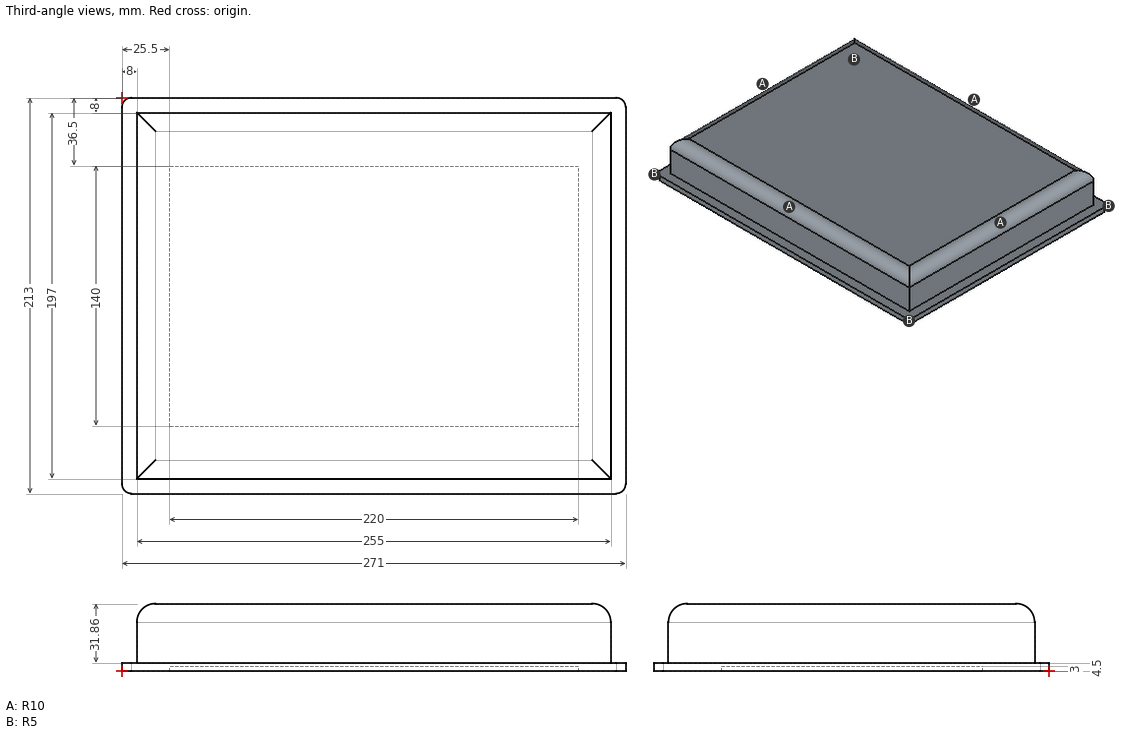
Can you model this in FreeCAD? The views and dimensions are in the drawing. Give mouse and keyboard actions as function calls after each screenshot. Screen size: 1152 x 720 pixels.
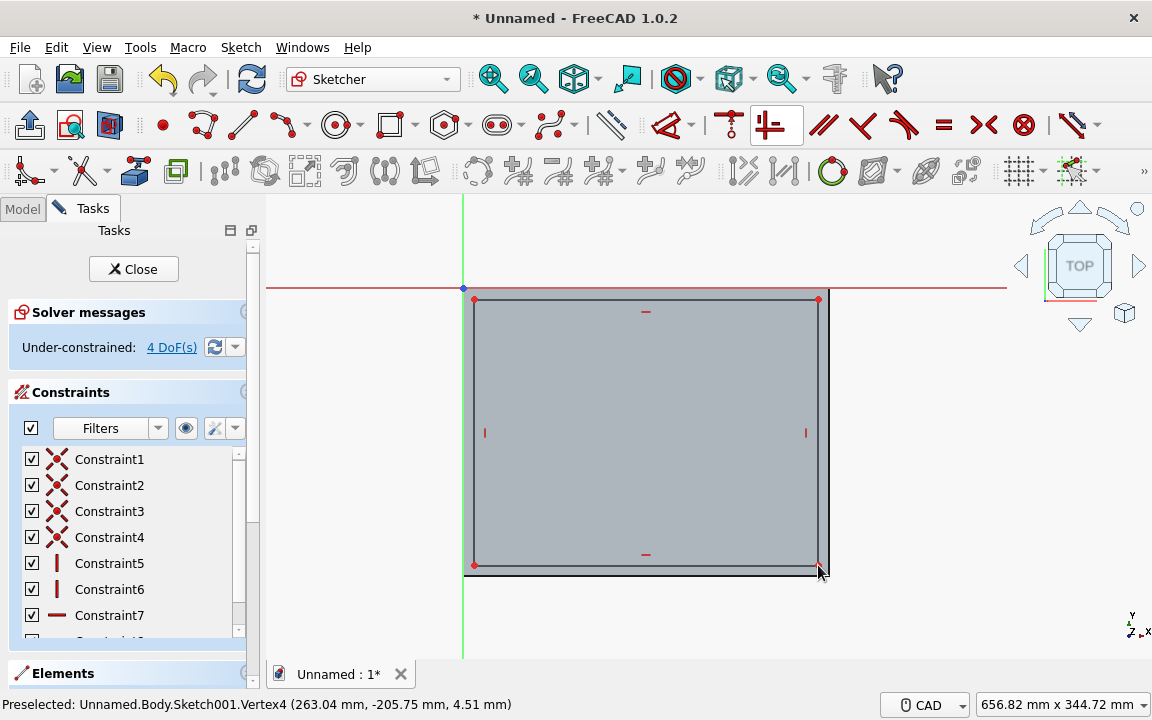
click(666, 126)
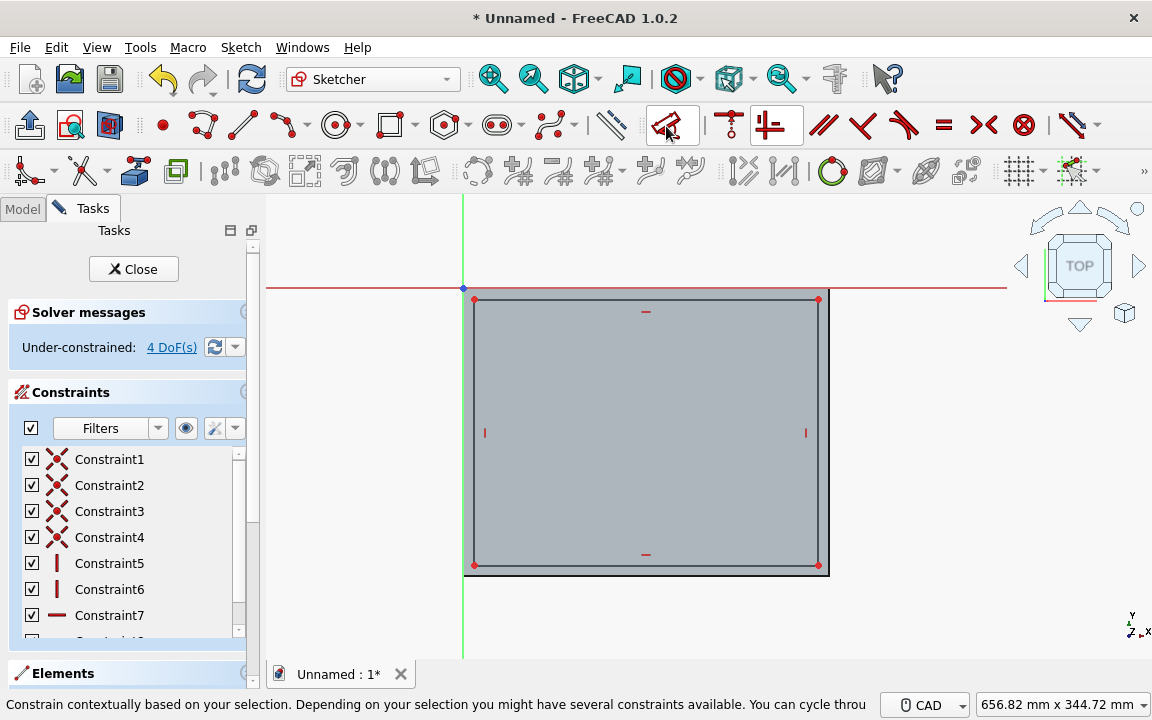
scroll(474, 300, up, 7)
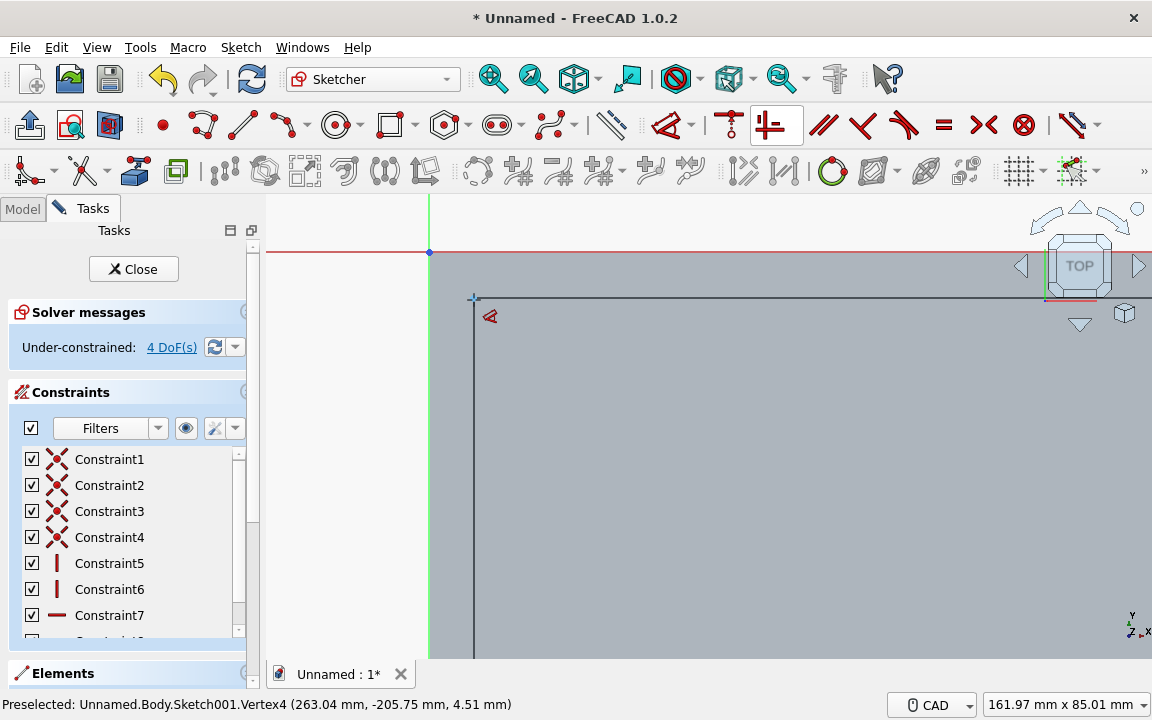
click(474, 298)
click(451, 332)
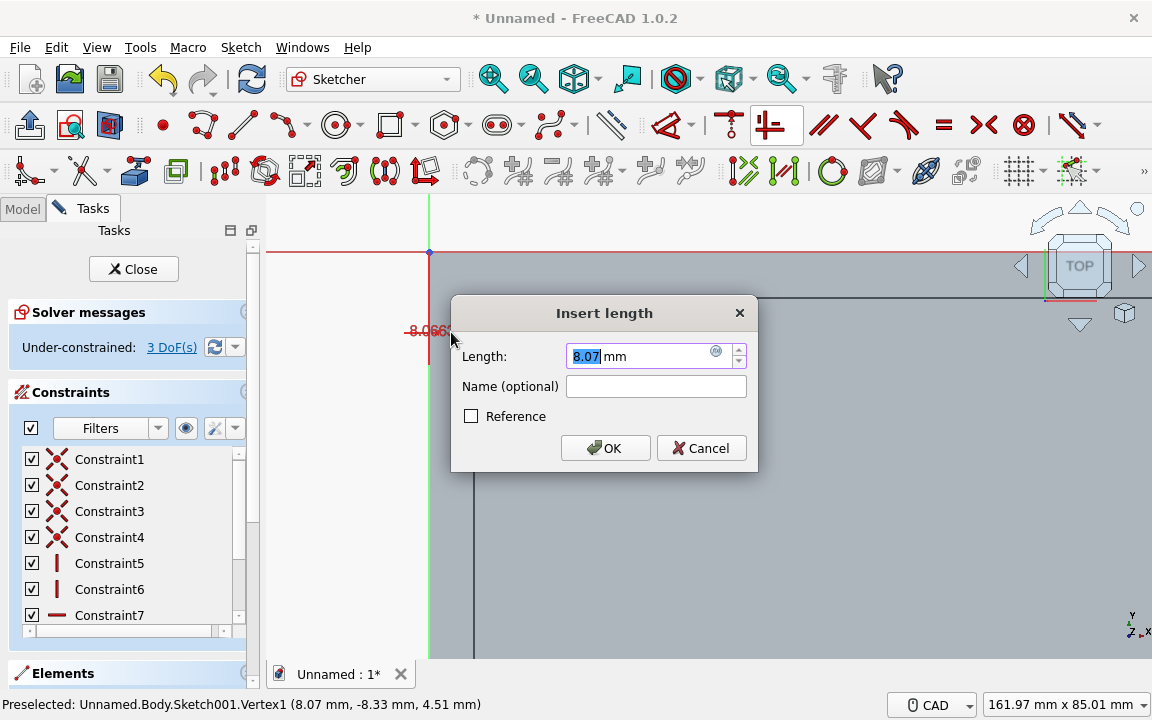
text(8)
key(Return)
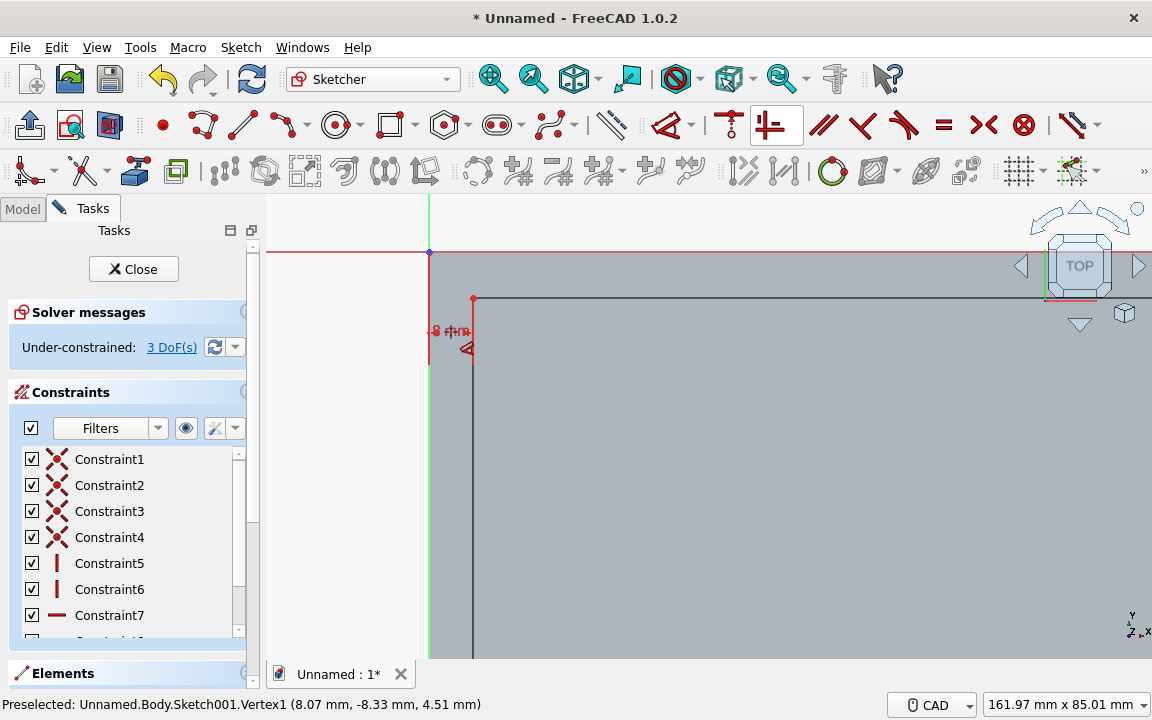
click(473, 298)
click(395, 275)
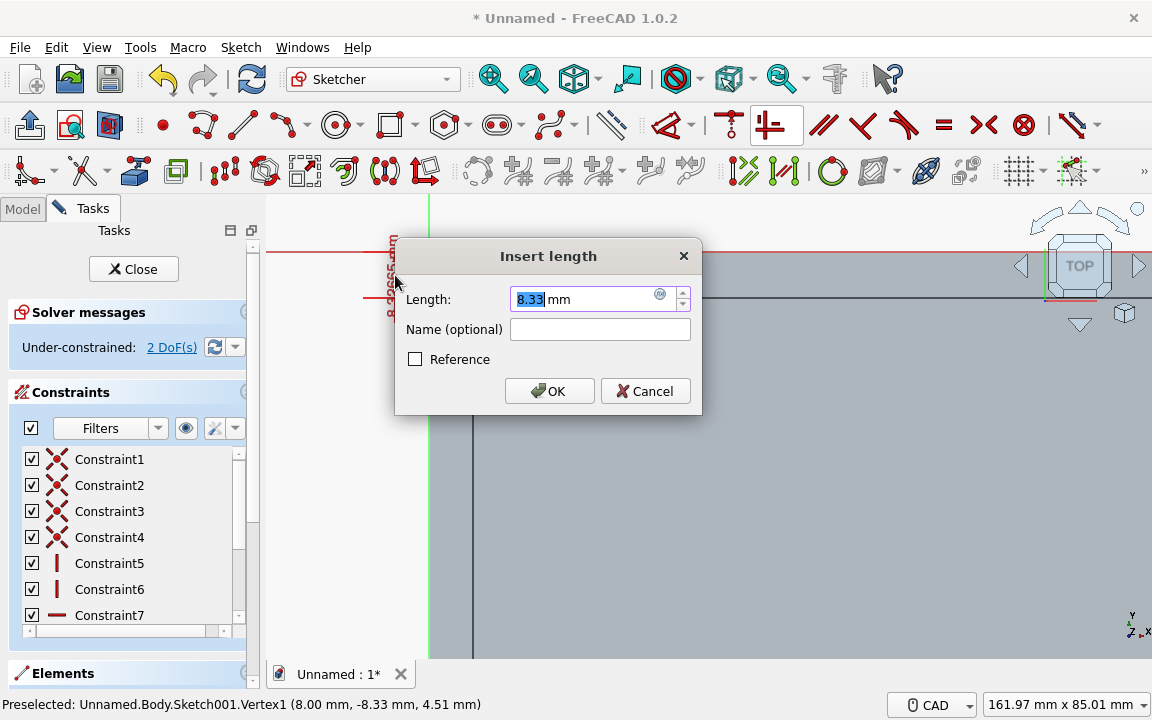
text(8)
key(Return)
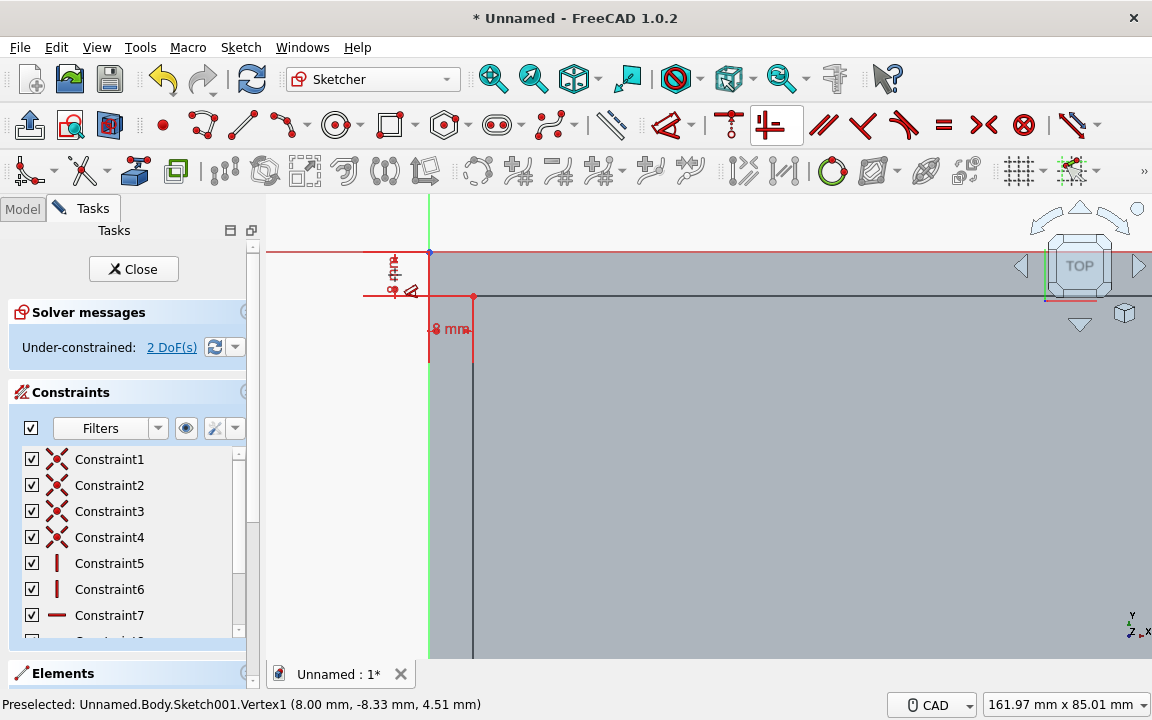
scroll(474, 300, down, 7)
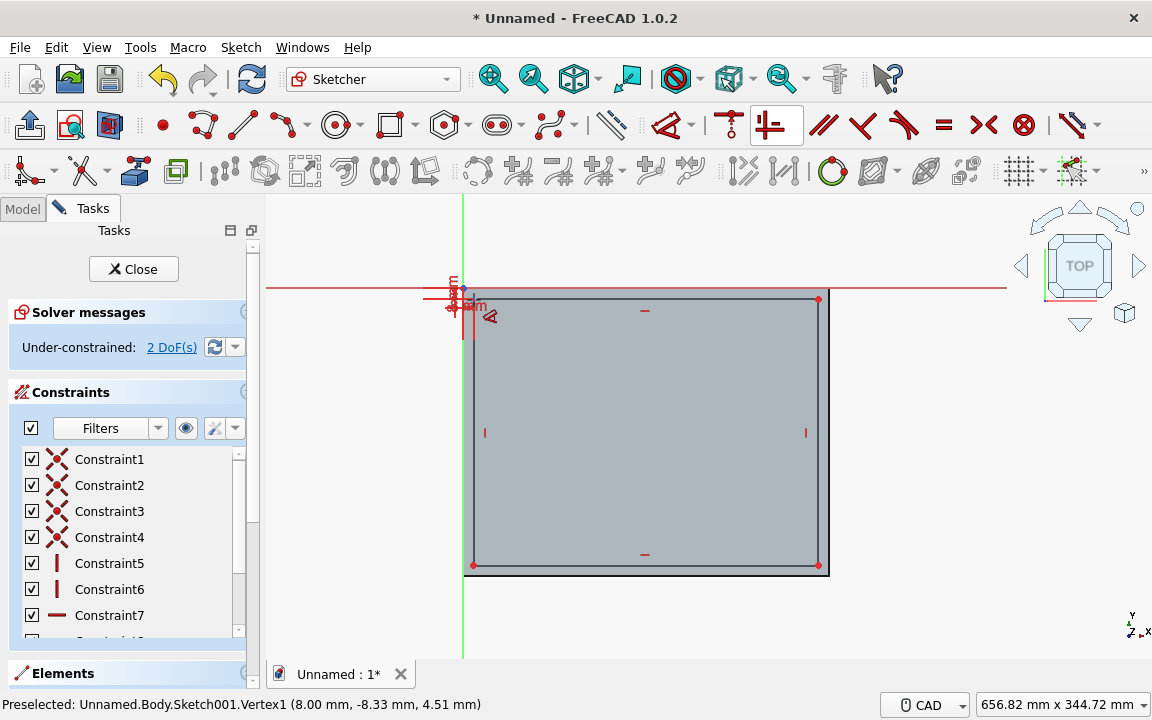
scroll(474, 379, up, 2)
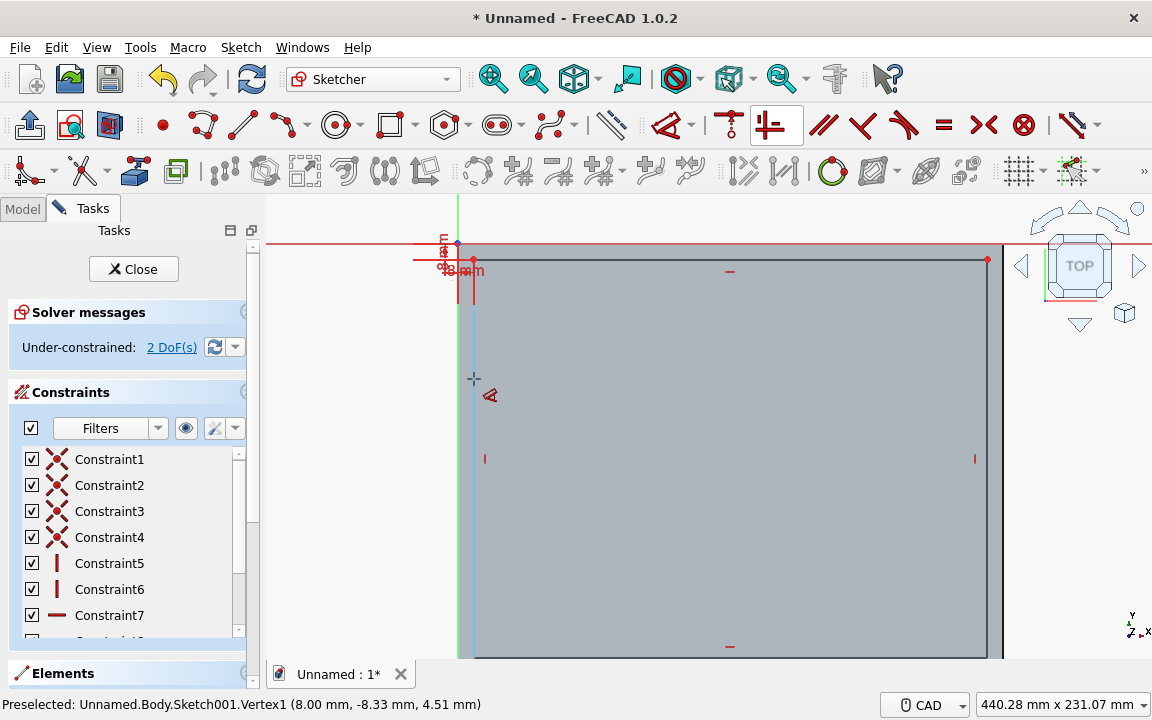
click(474, 379)
click(440, 445)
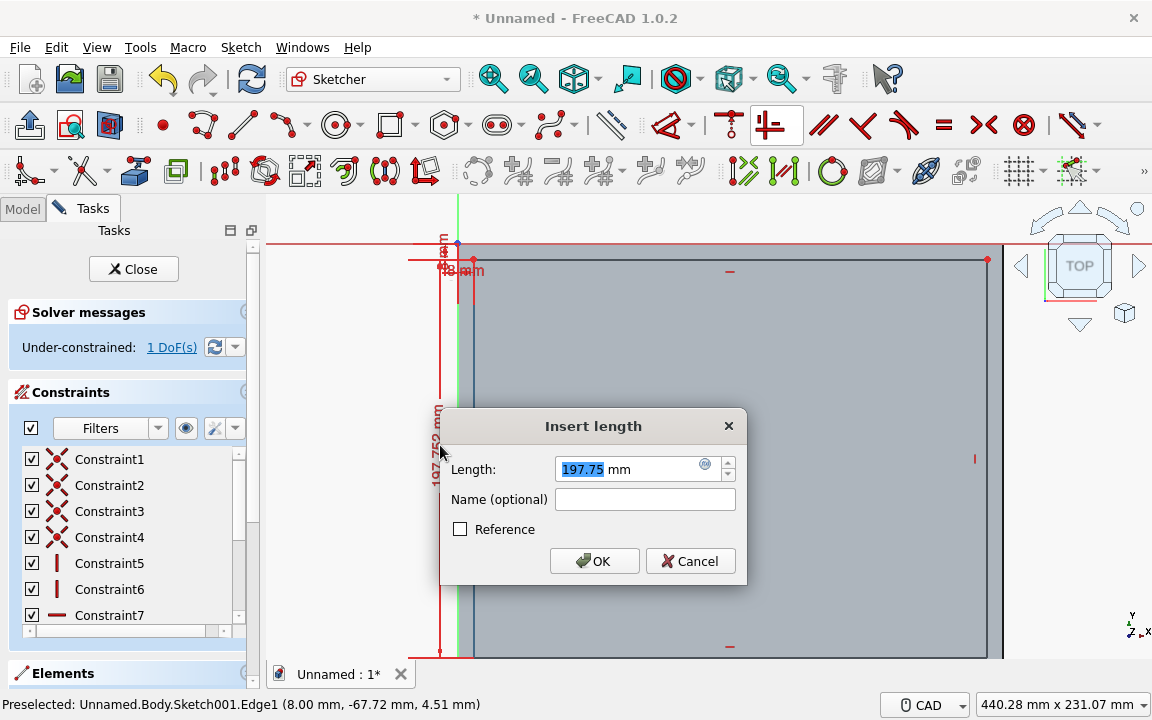
text(197)
key(Return)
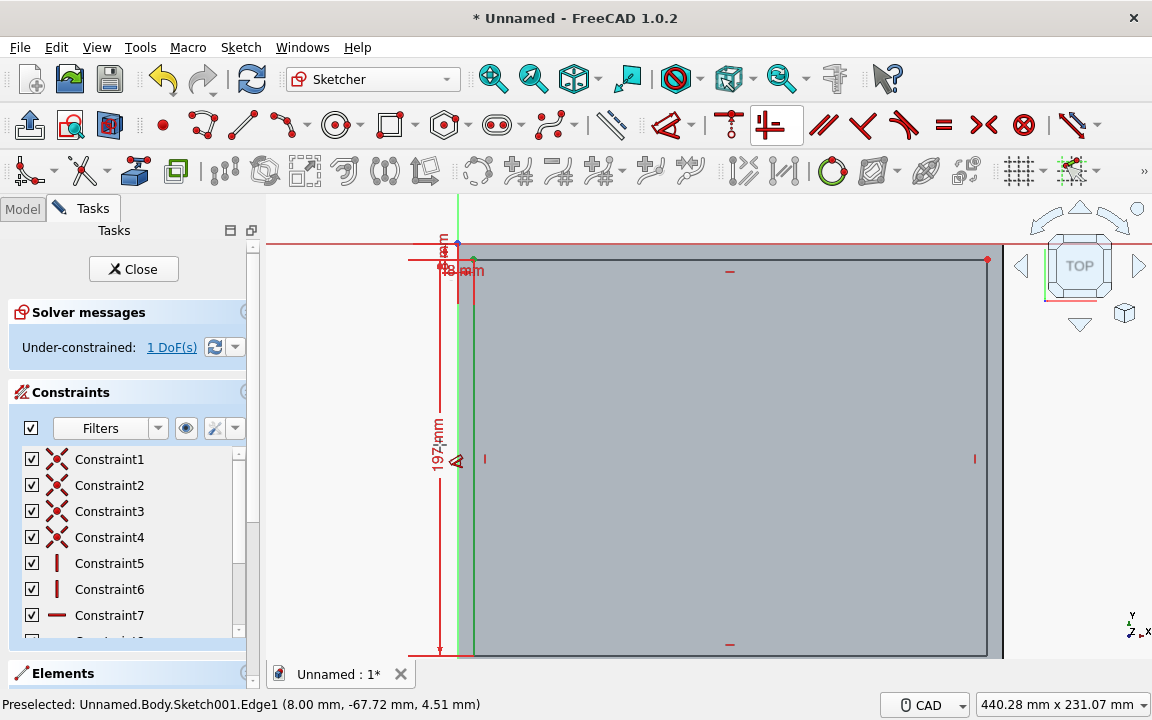
scroll(474, 379, down, 2)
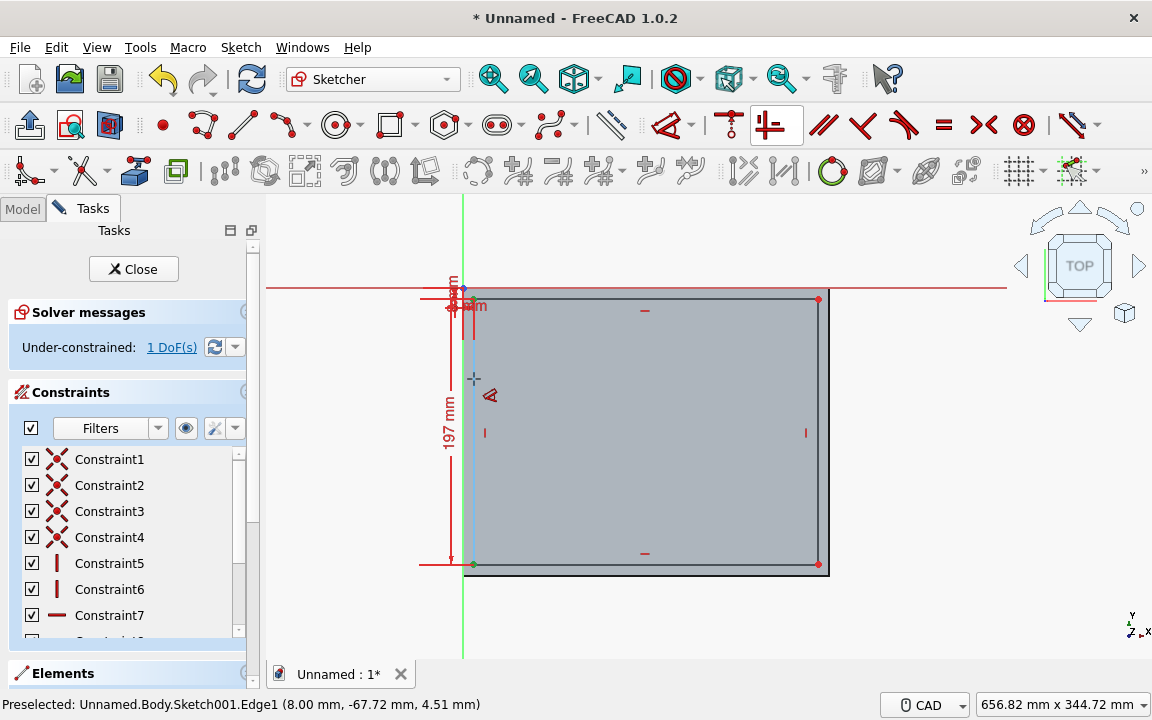
click(577, 565)
click(646, 599)